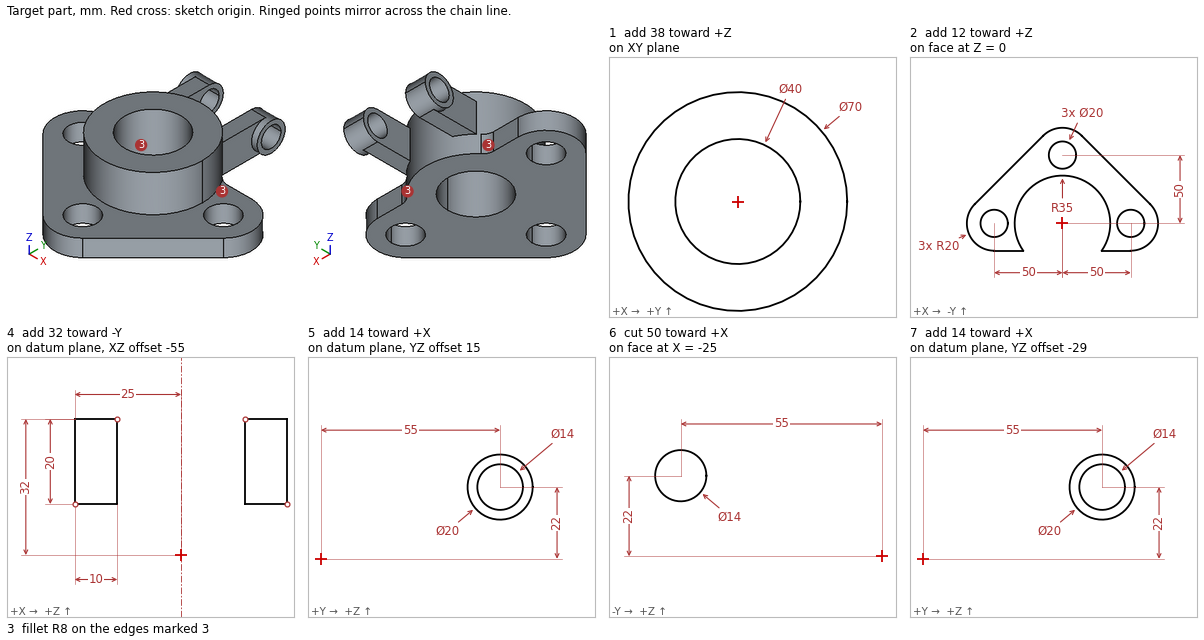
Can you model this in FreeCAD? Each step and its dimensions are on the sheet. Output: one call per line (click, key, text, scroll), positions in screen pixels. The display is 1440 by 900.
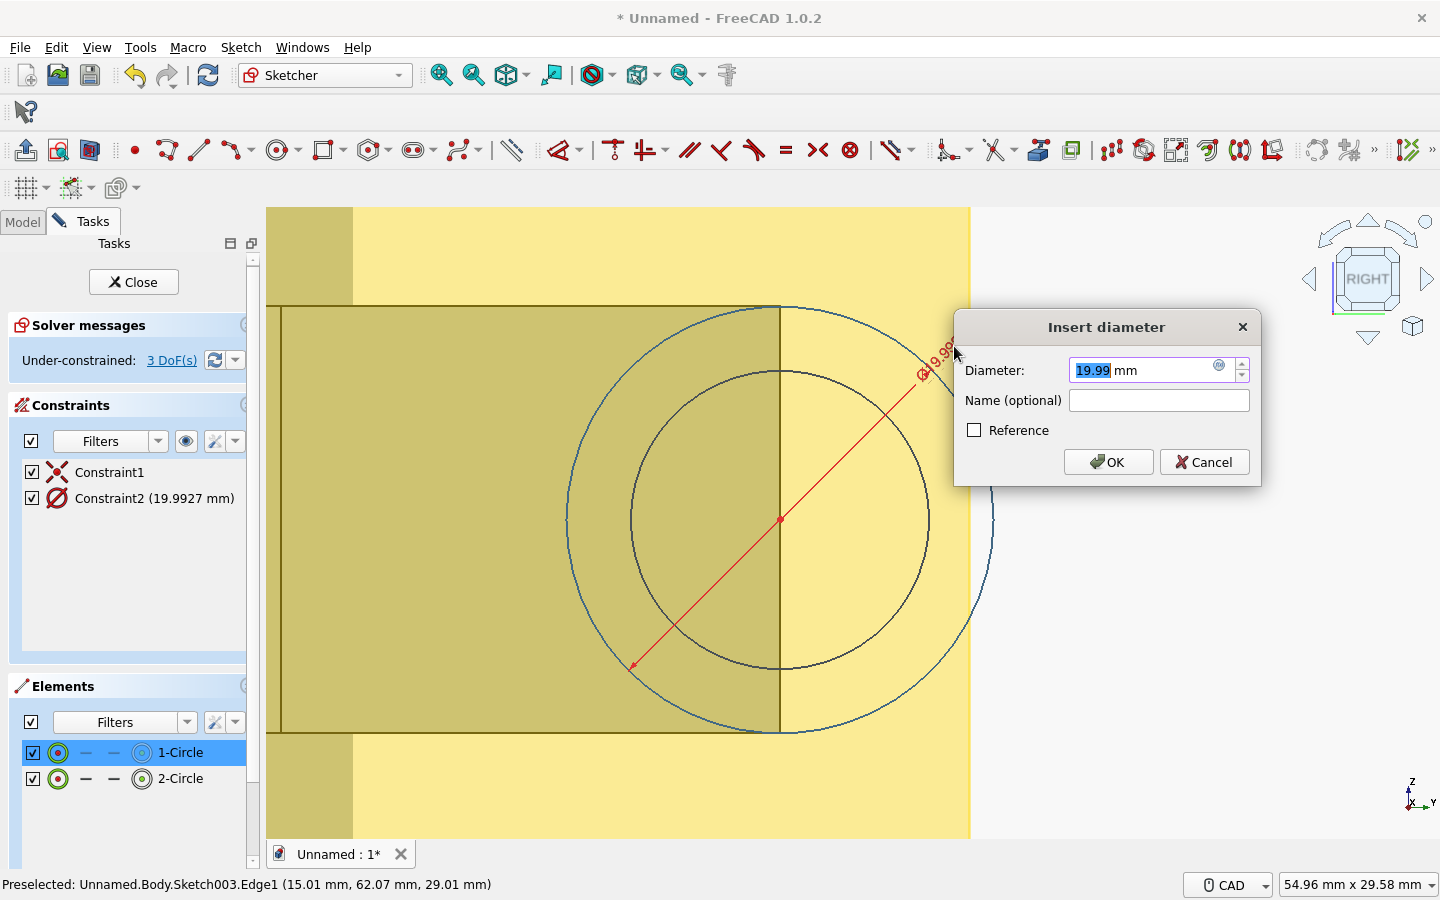
text(20)
key(Return)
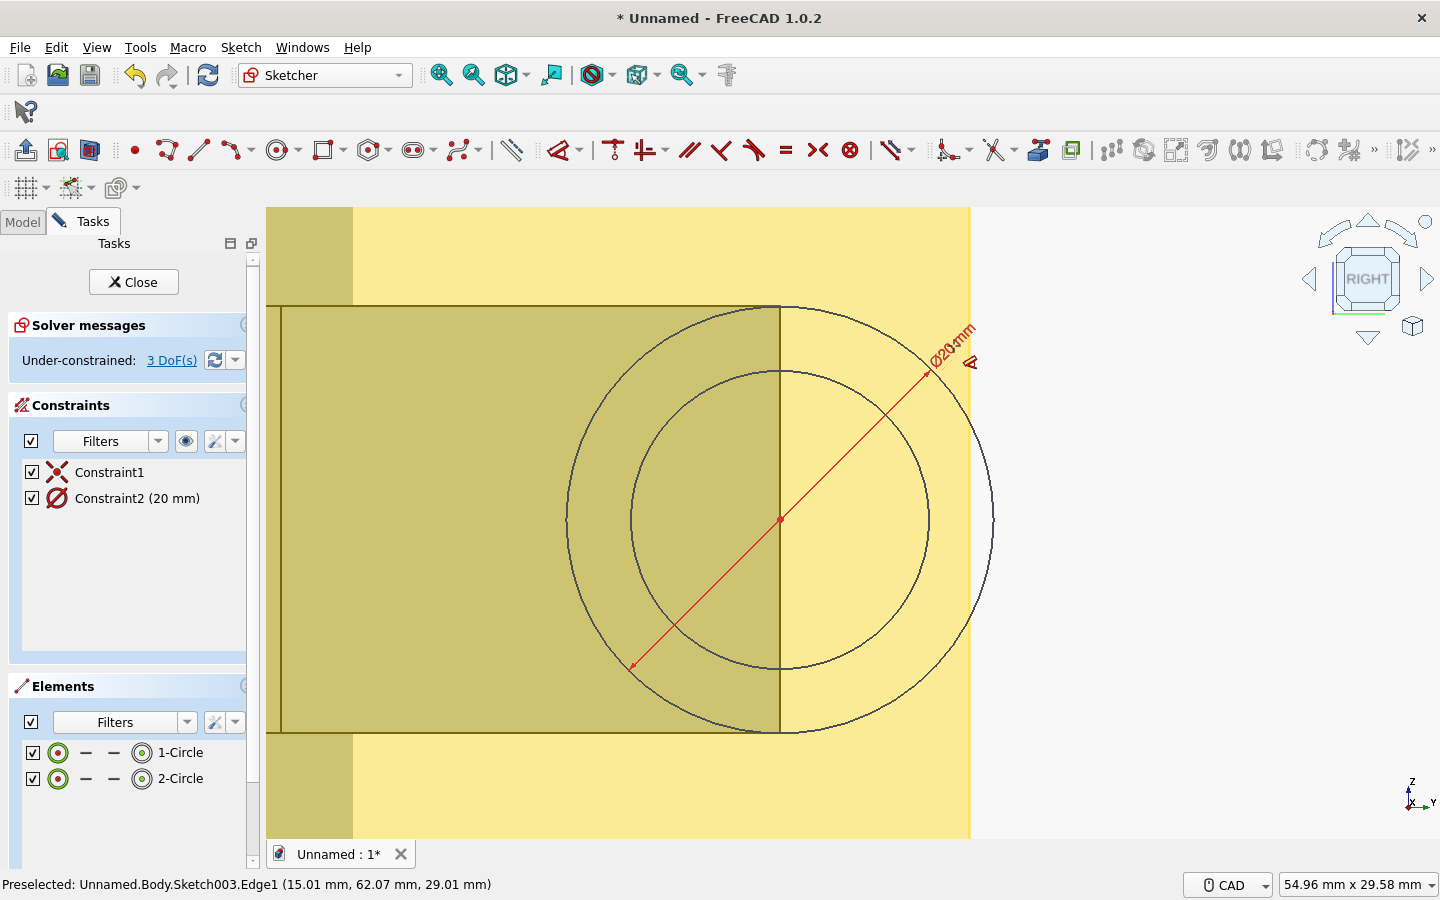
click(885, 414)
click(908, 391)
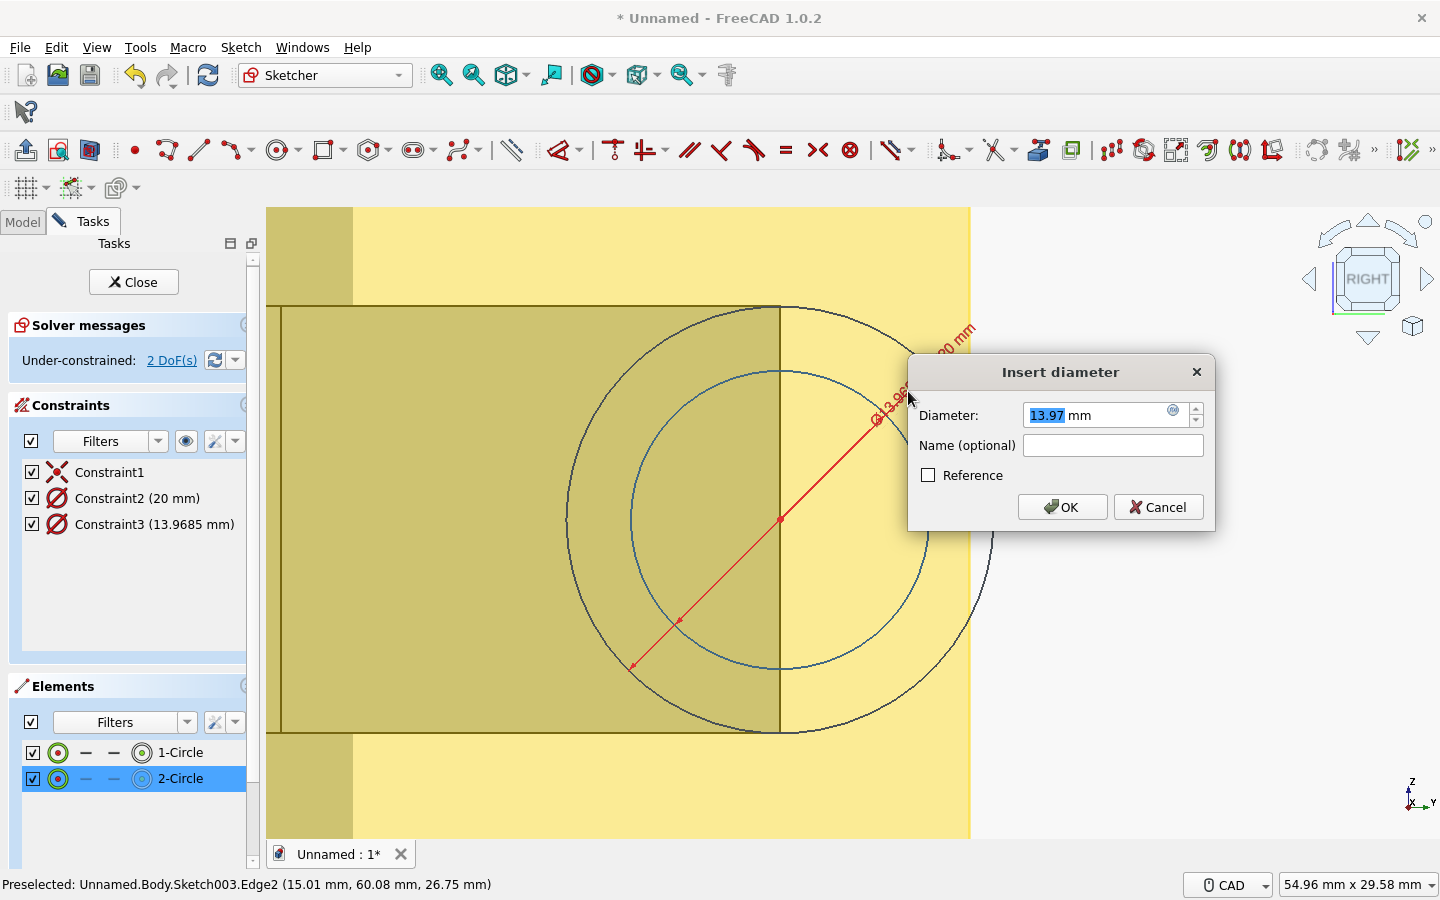
text(14)
key(Return)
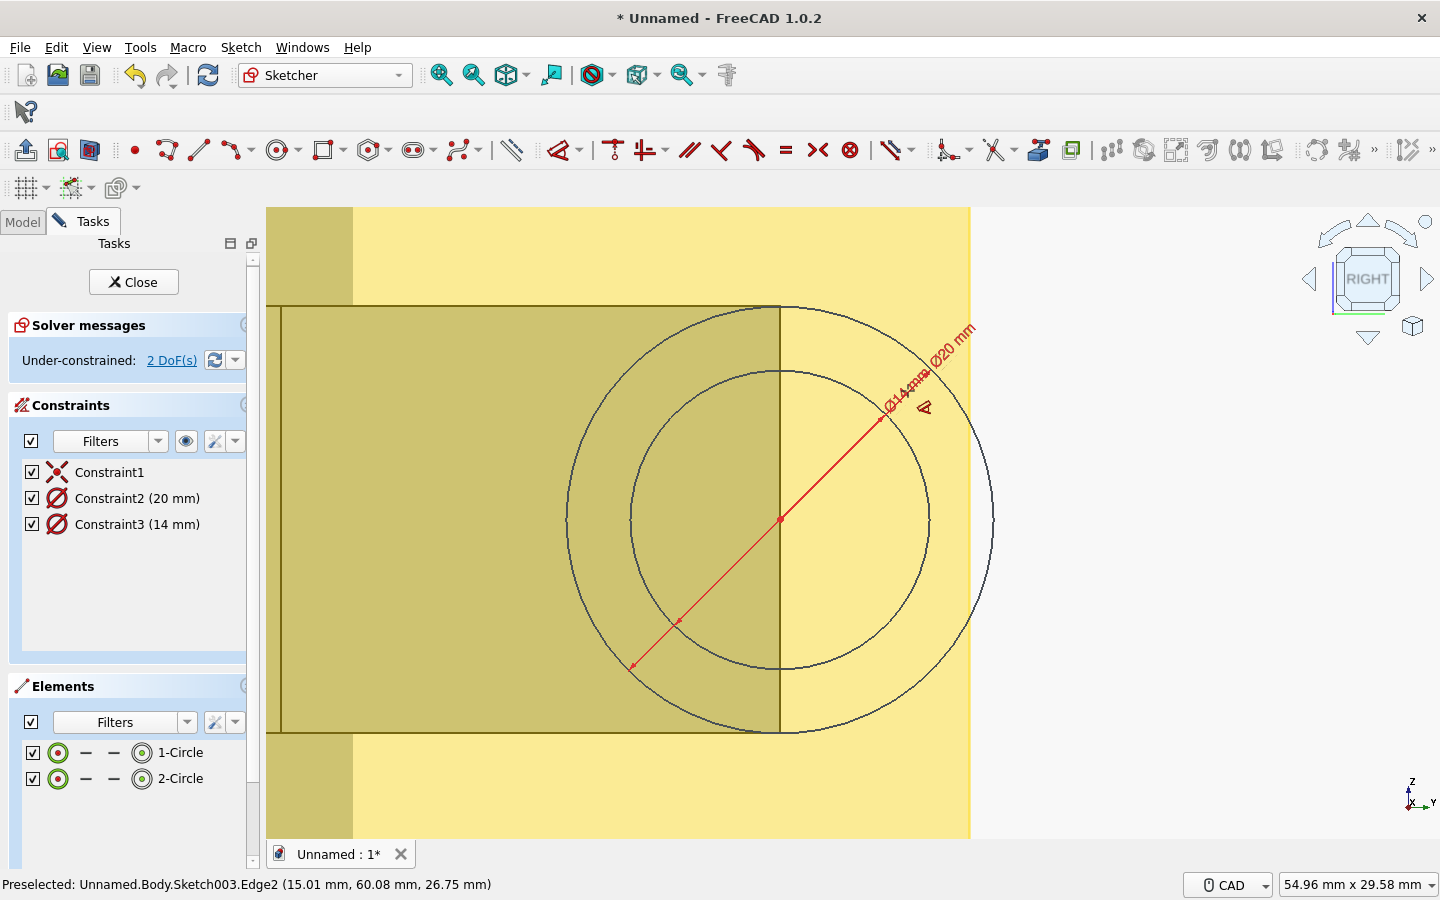
click(780, 520)
click(537, 486)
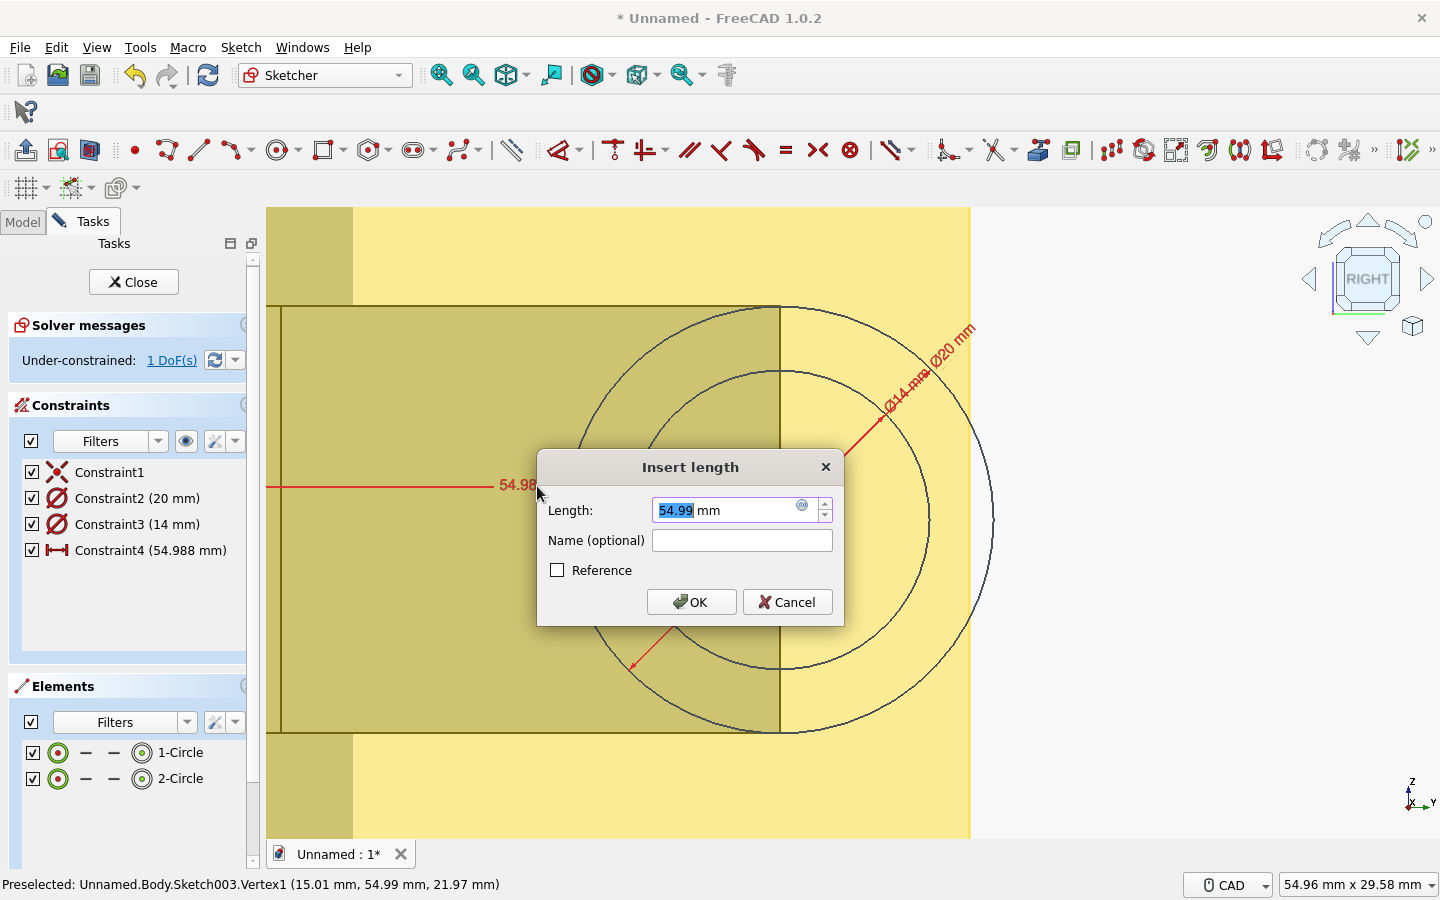
text(55)
key(Return)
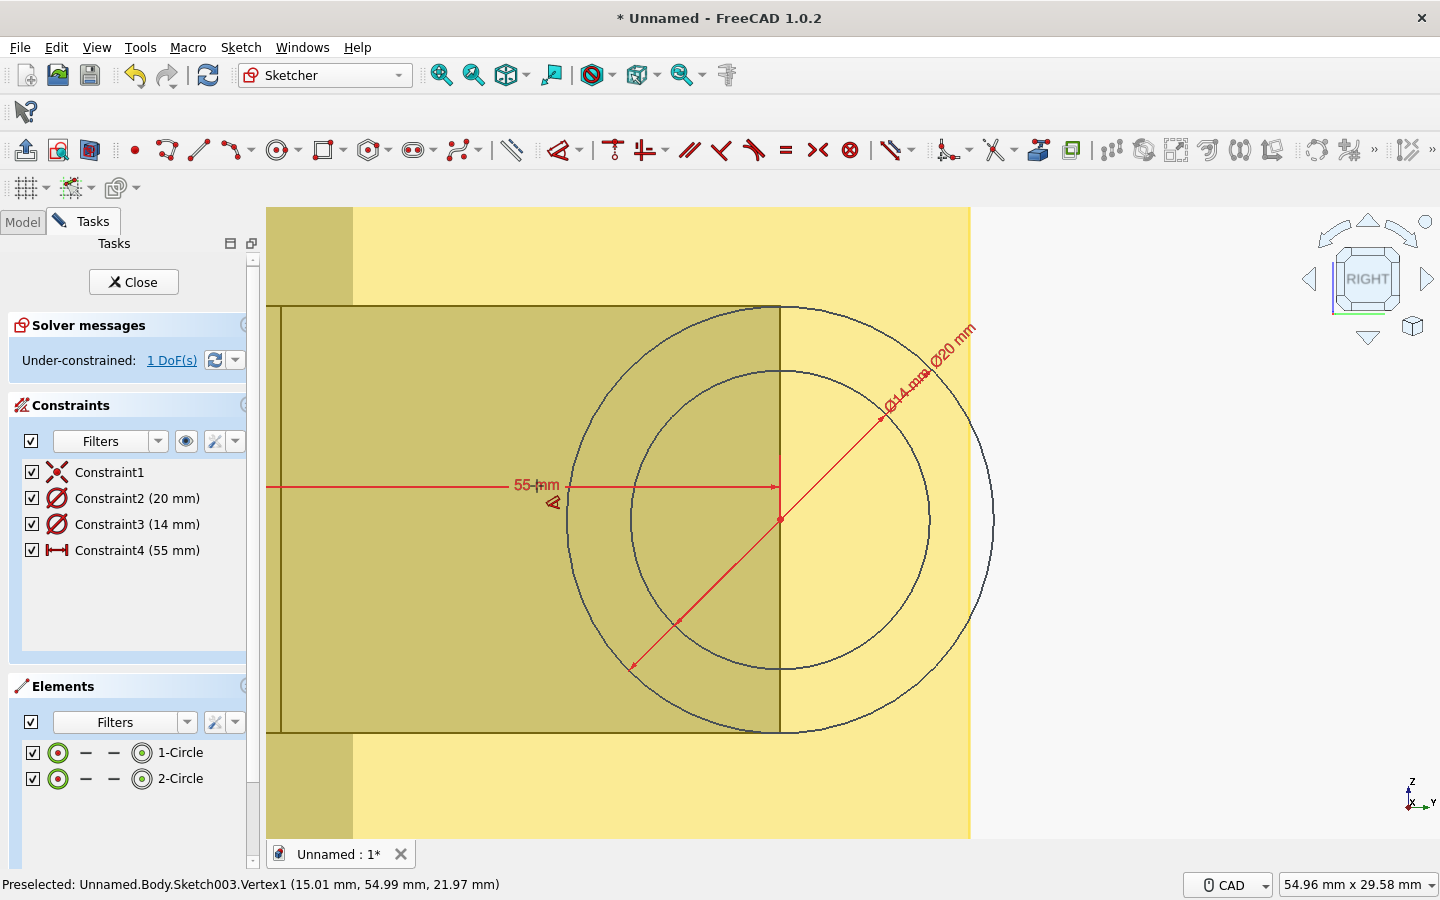
click(780, 520)
click(814, 599)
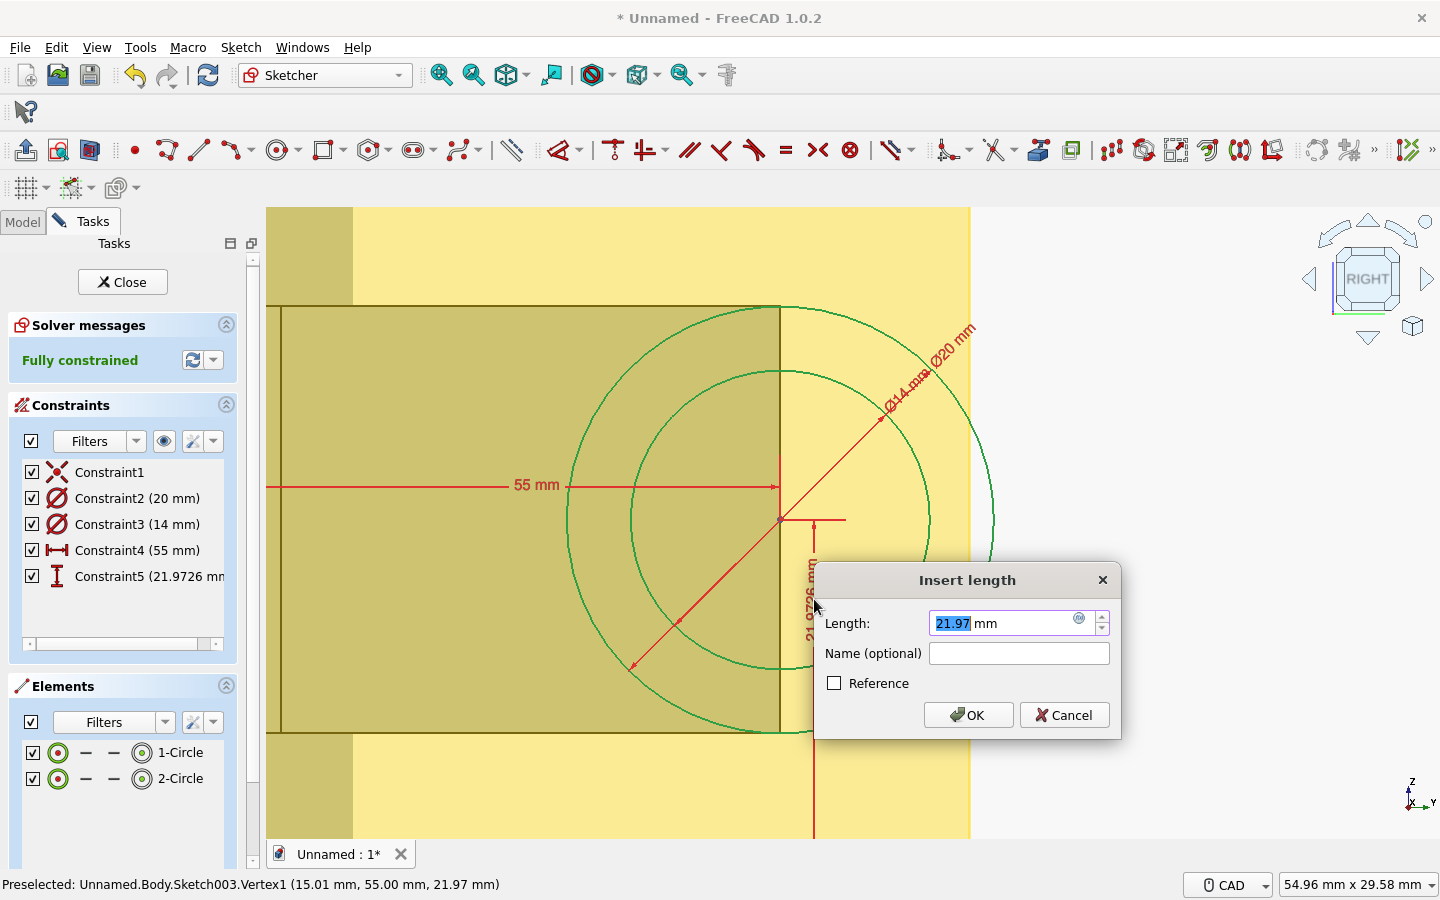
text(22)
key(Return)
key(Escape)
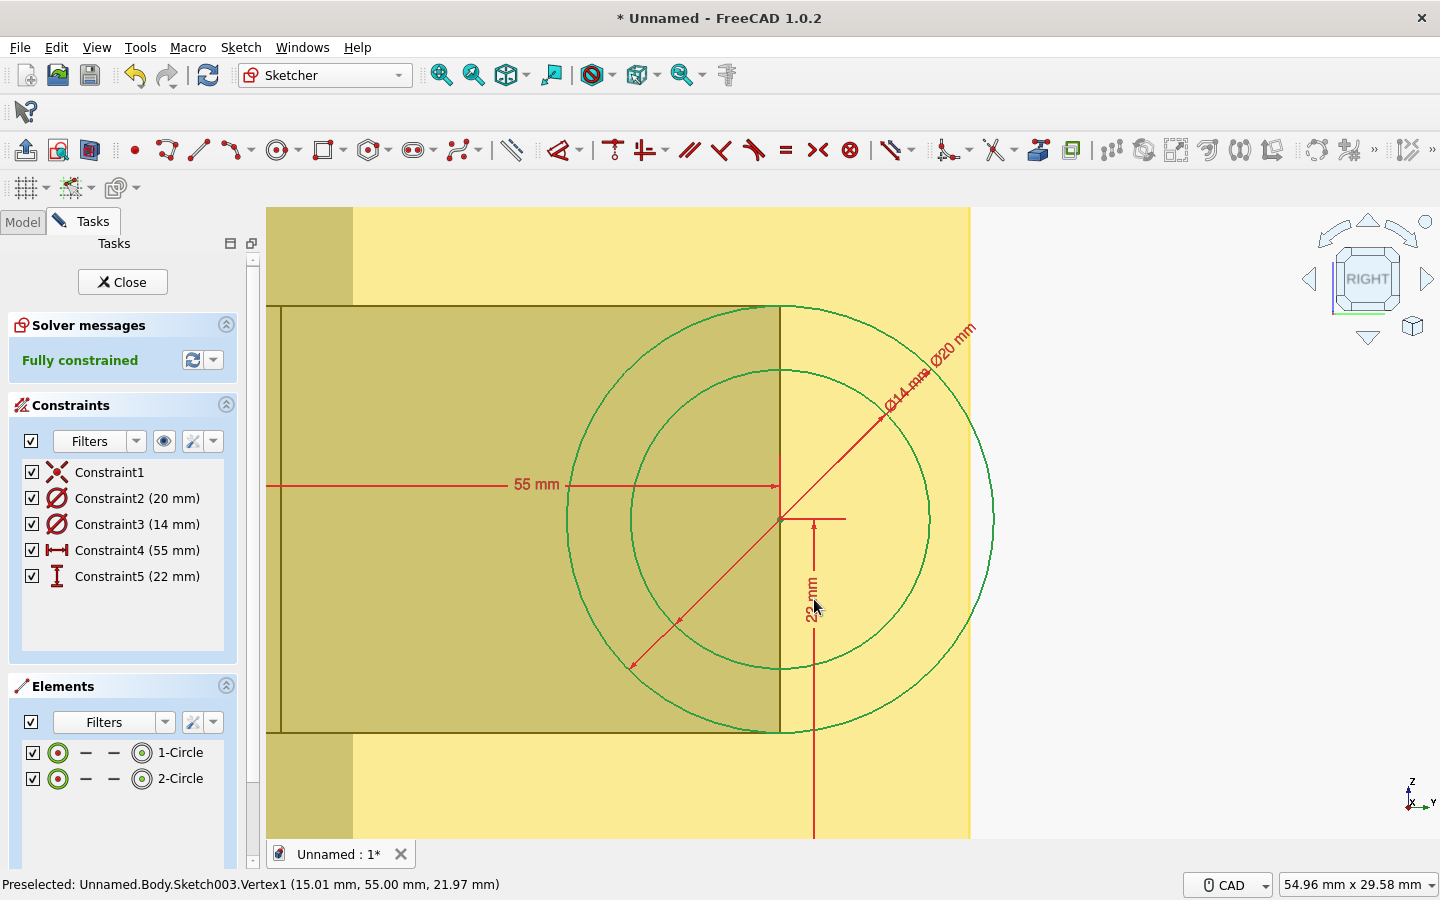
click(123, 282)